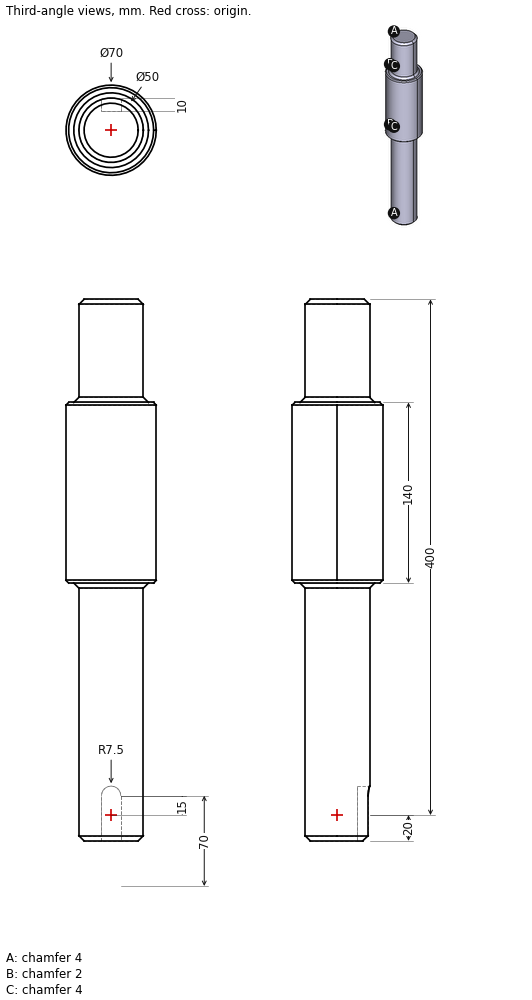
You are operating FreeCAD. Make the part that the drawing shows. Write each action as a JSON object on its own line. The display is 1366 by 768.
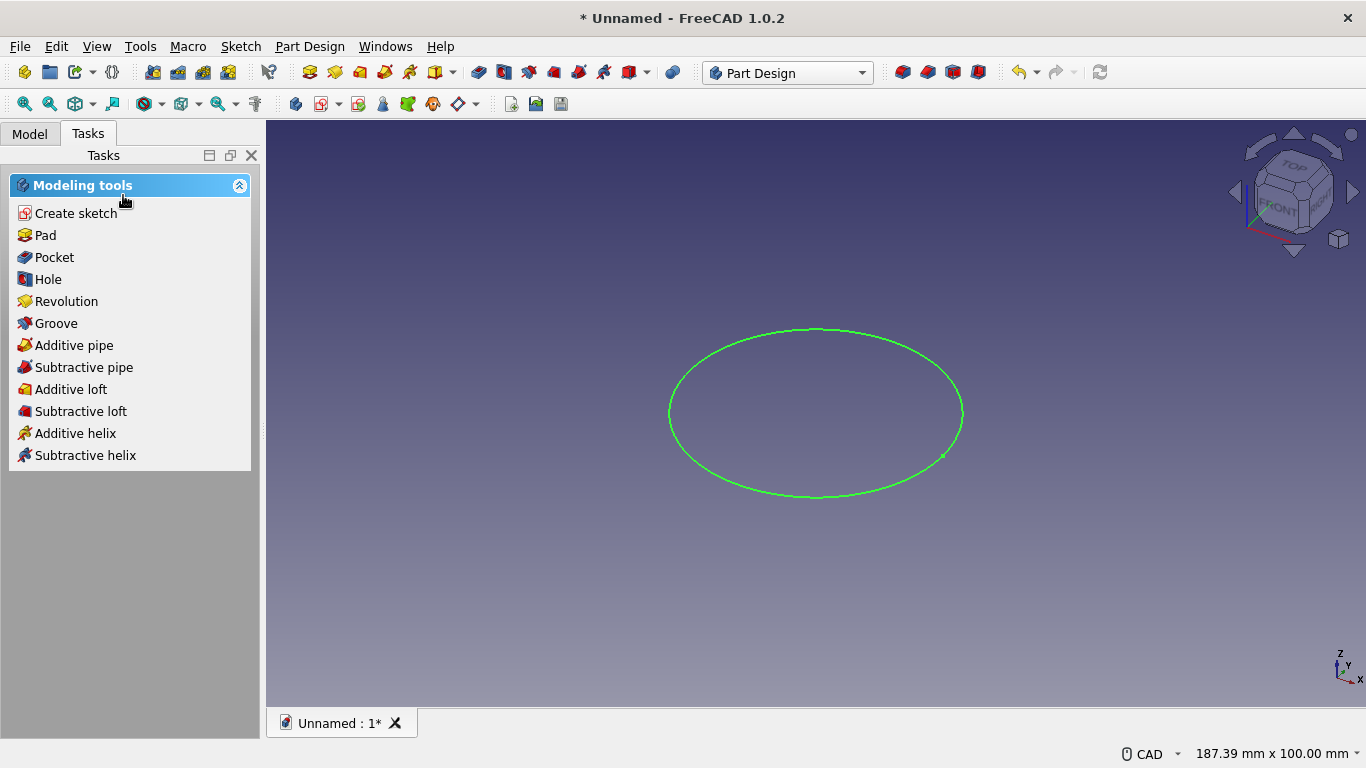
{"action": "left_click", "coordinate": [310, 72]}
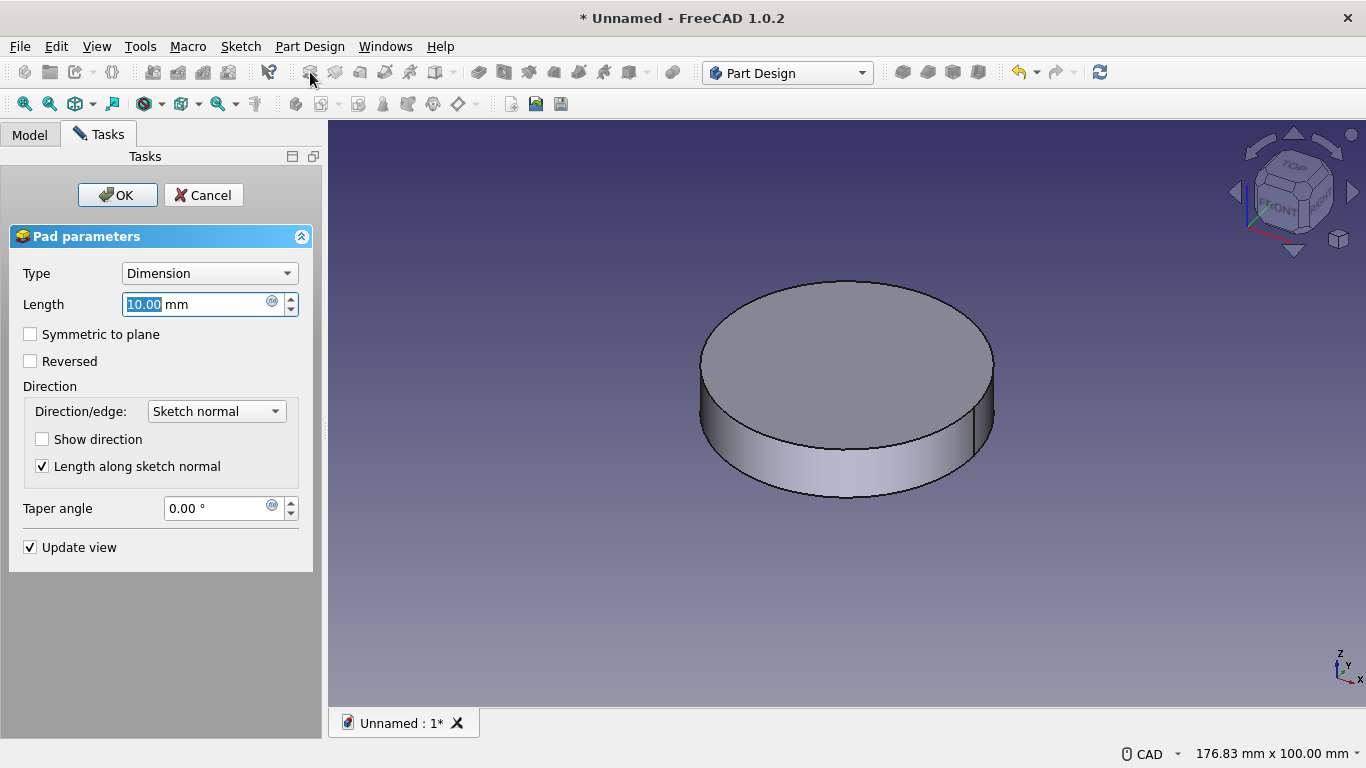
{"action": "left_click", "coordinate": [210, 274]}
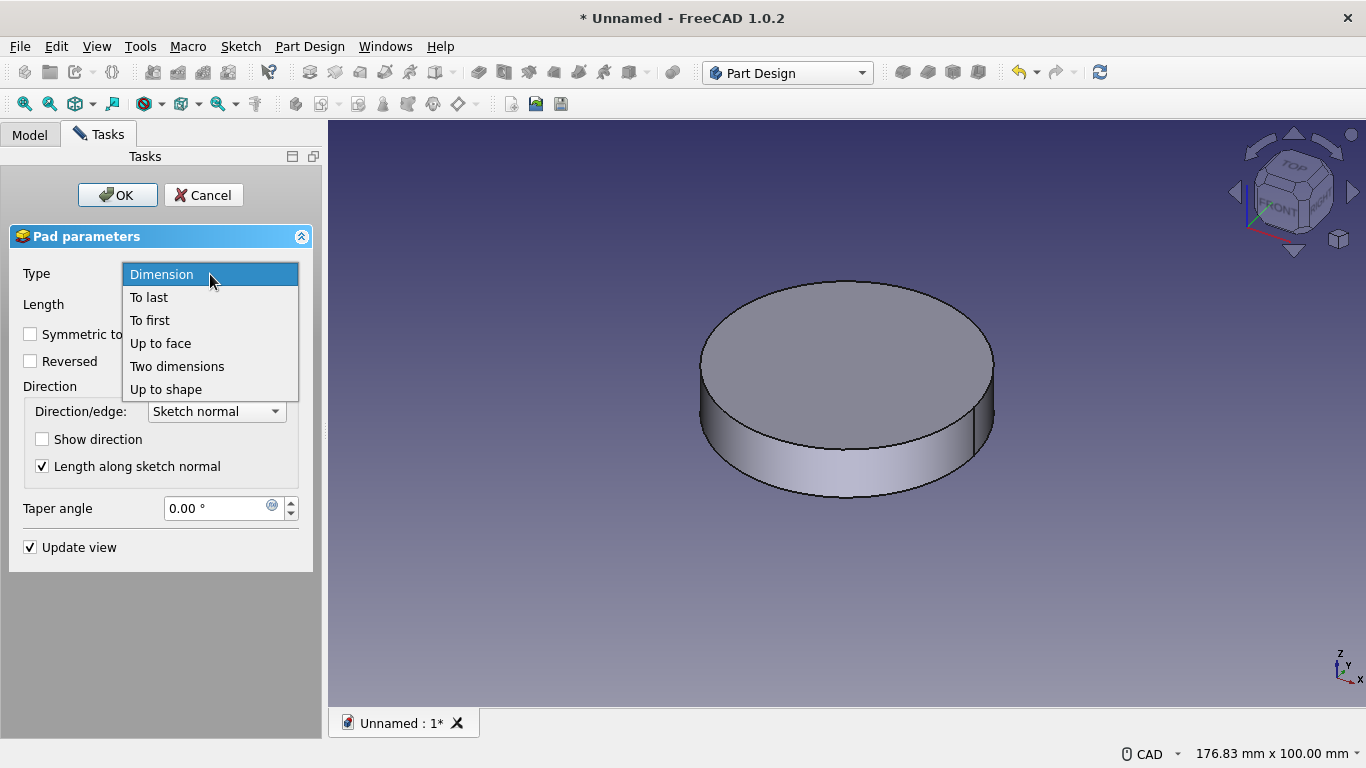
{"action": "left_click", "coordinate": [208, 366]}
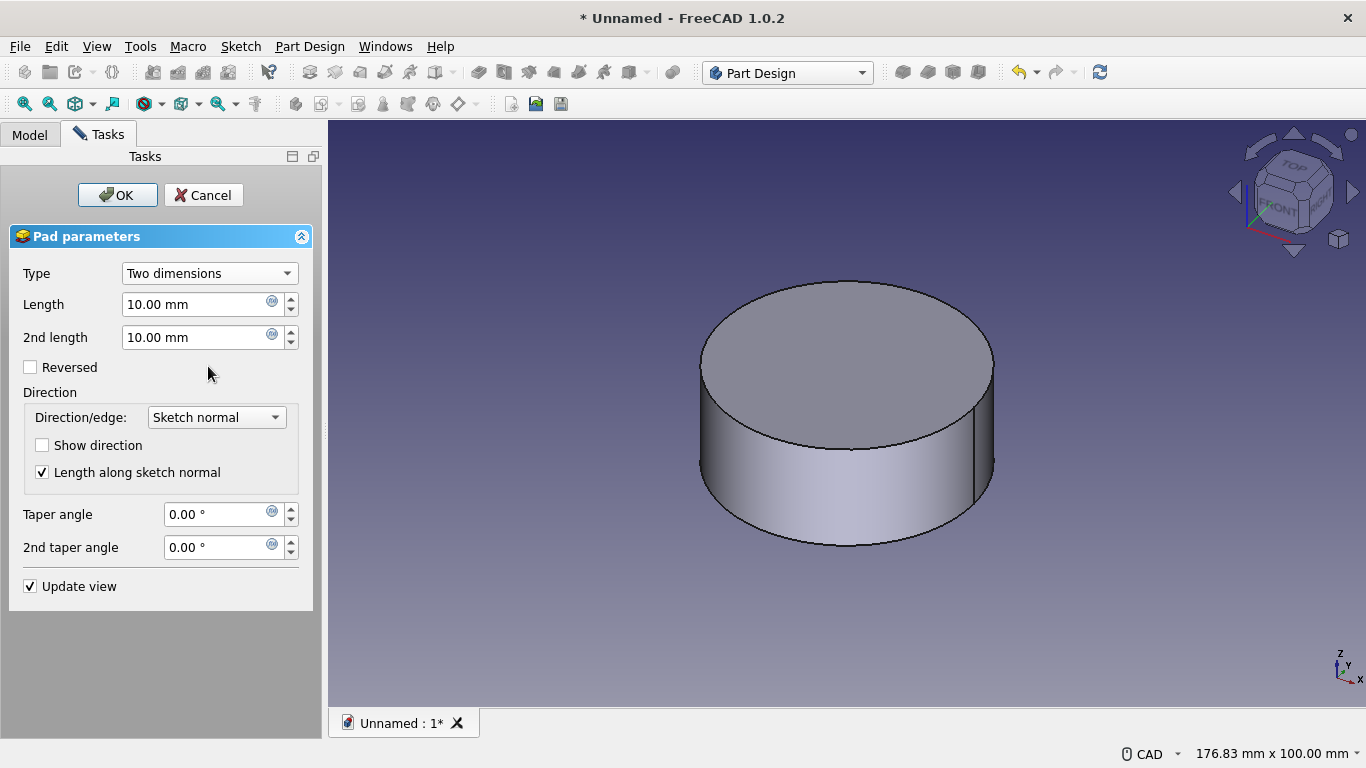
{"action": "triple_click", "coordinate": [204, 304]}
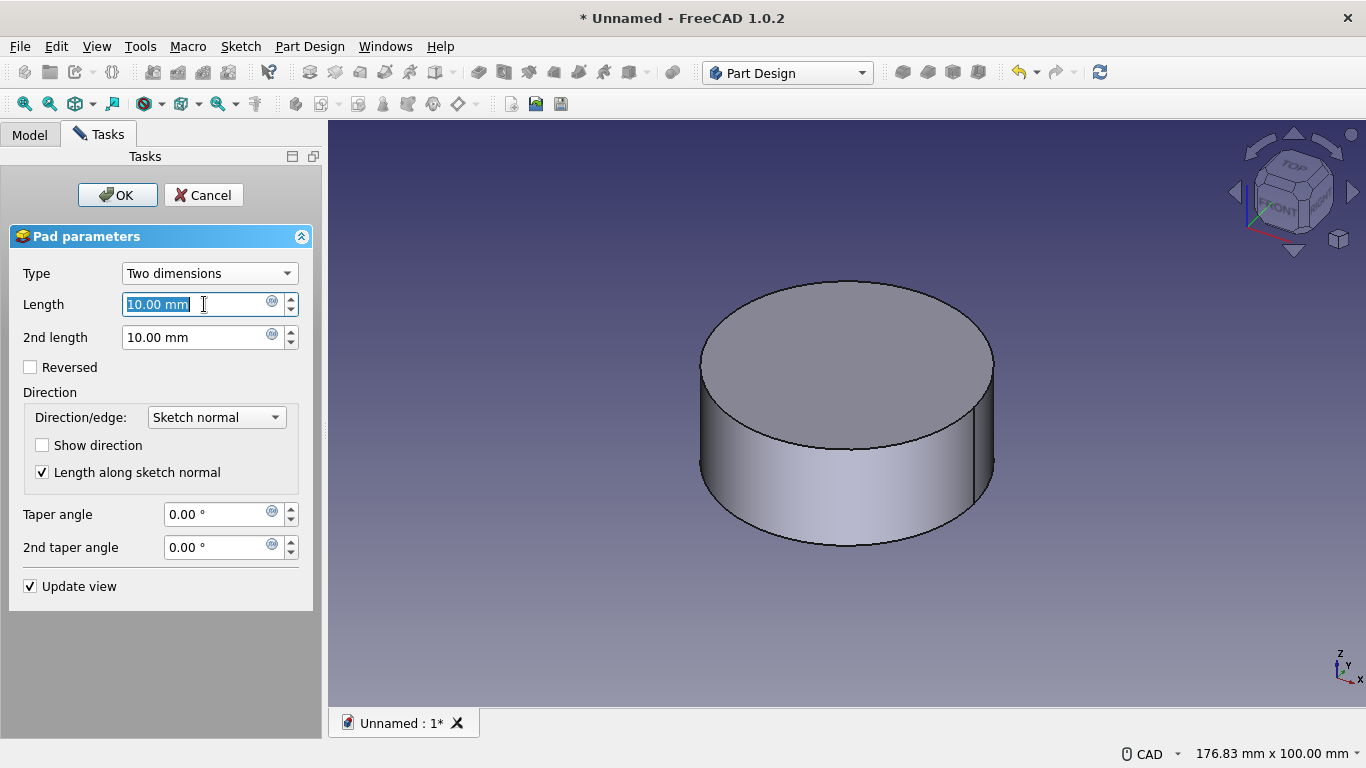
{"action": "type", "text": "400"}
{"action": "key", "text": "Tab"}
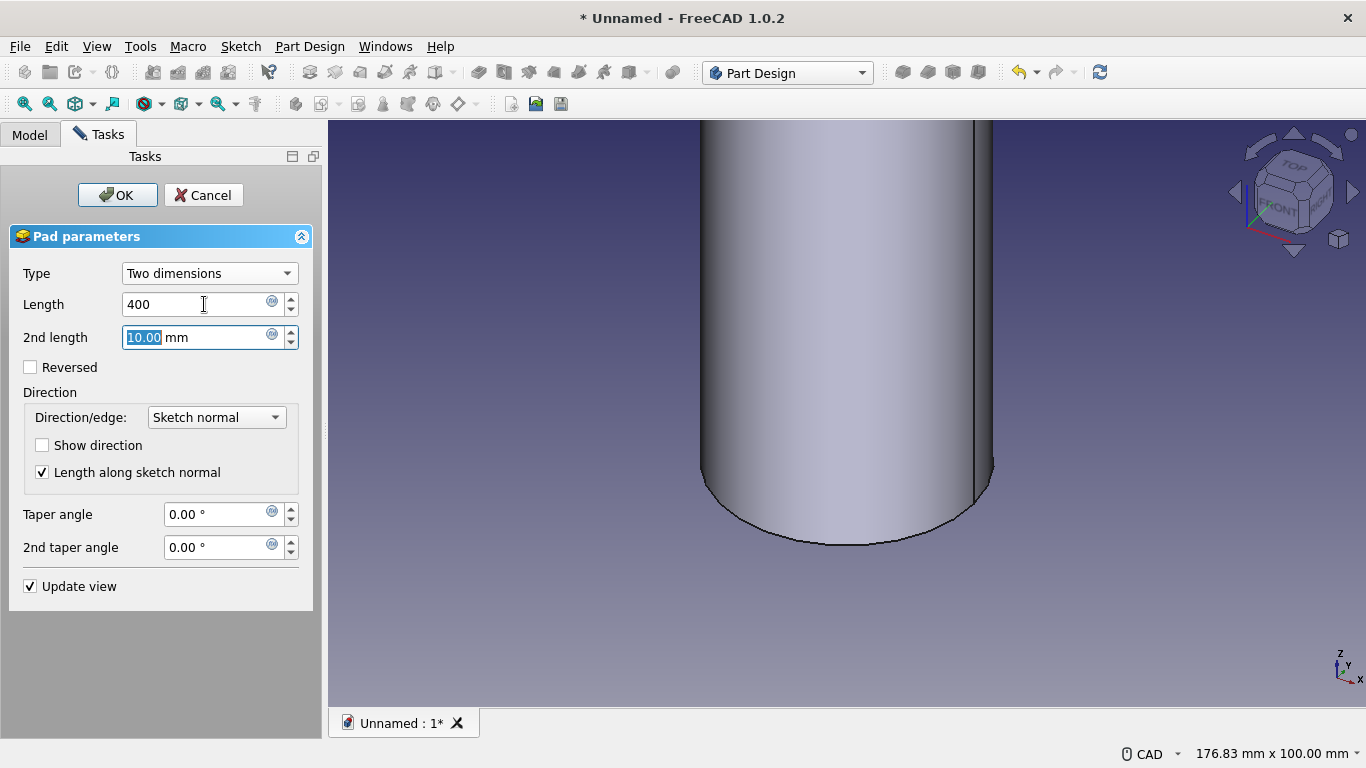
{"action": "type", "text": "20"}
{"action": "key", "text": "Tab"}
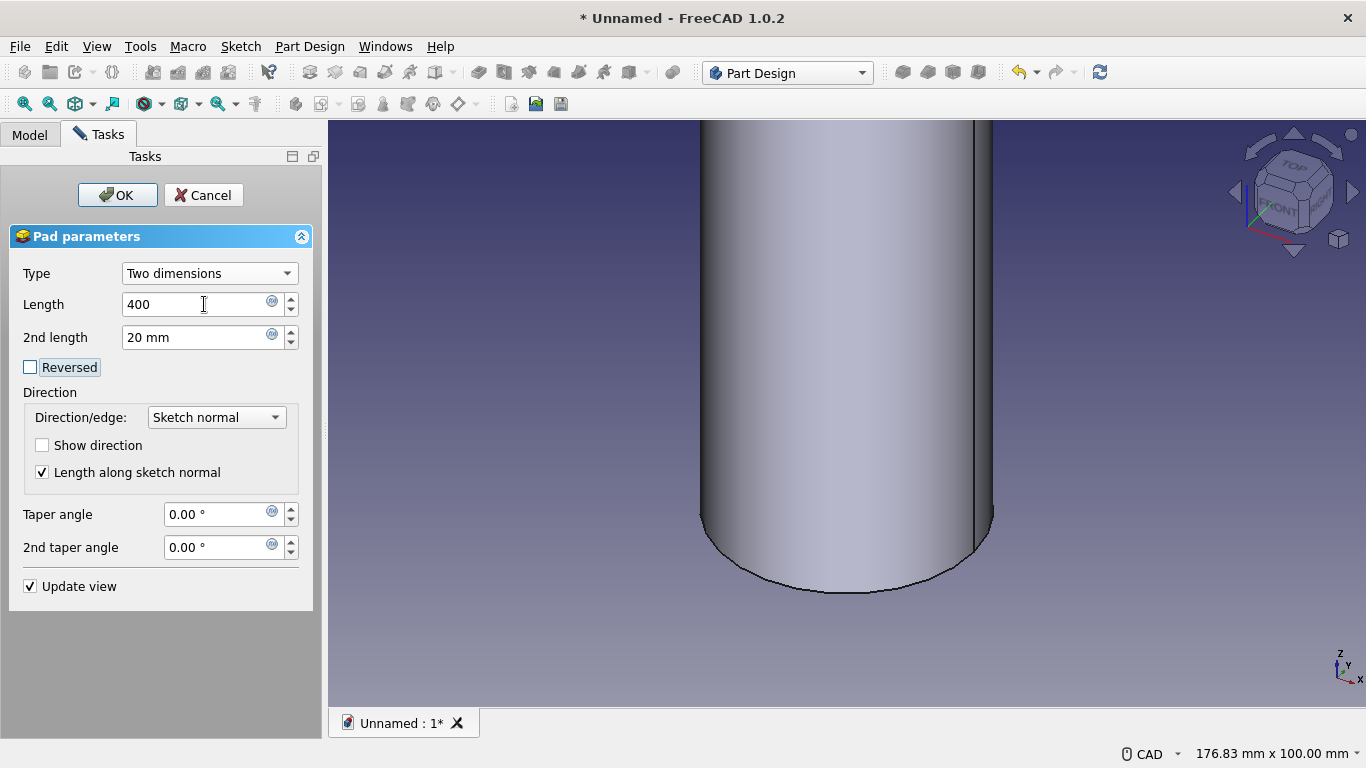
{"action": "left_click", "coordinate": [118, 195]}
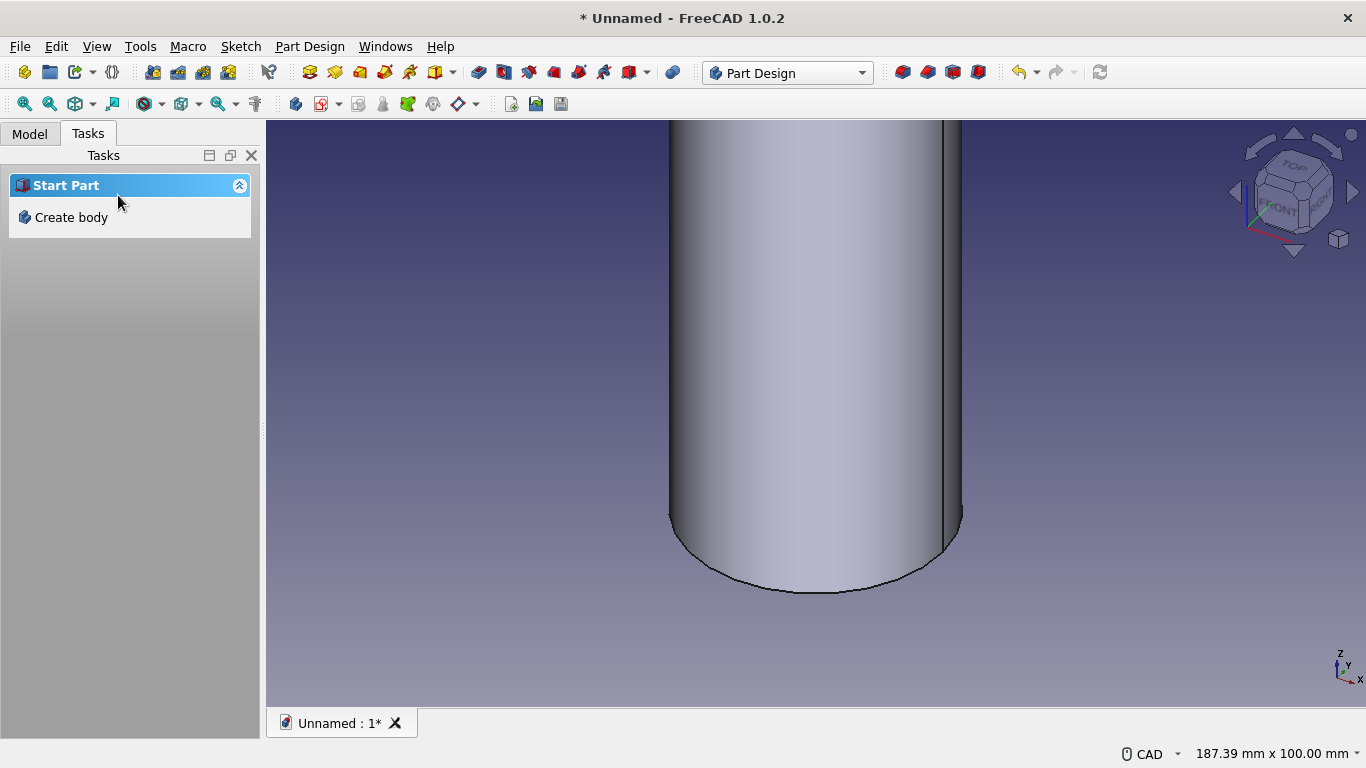
{"action": "left_click", "coordinate": [25, 104]}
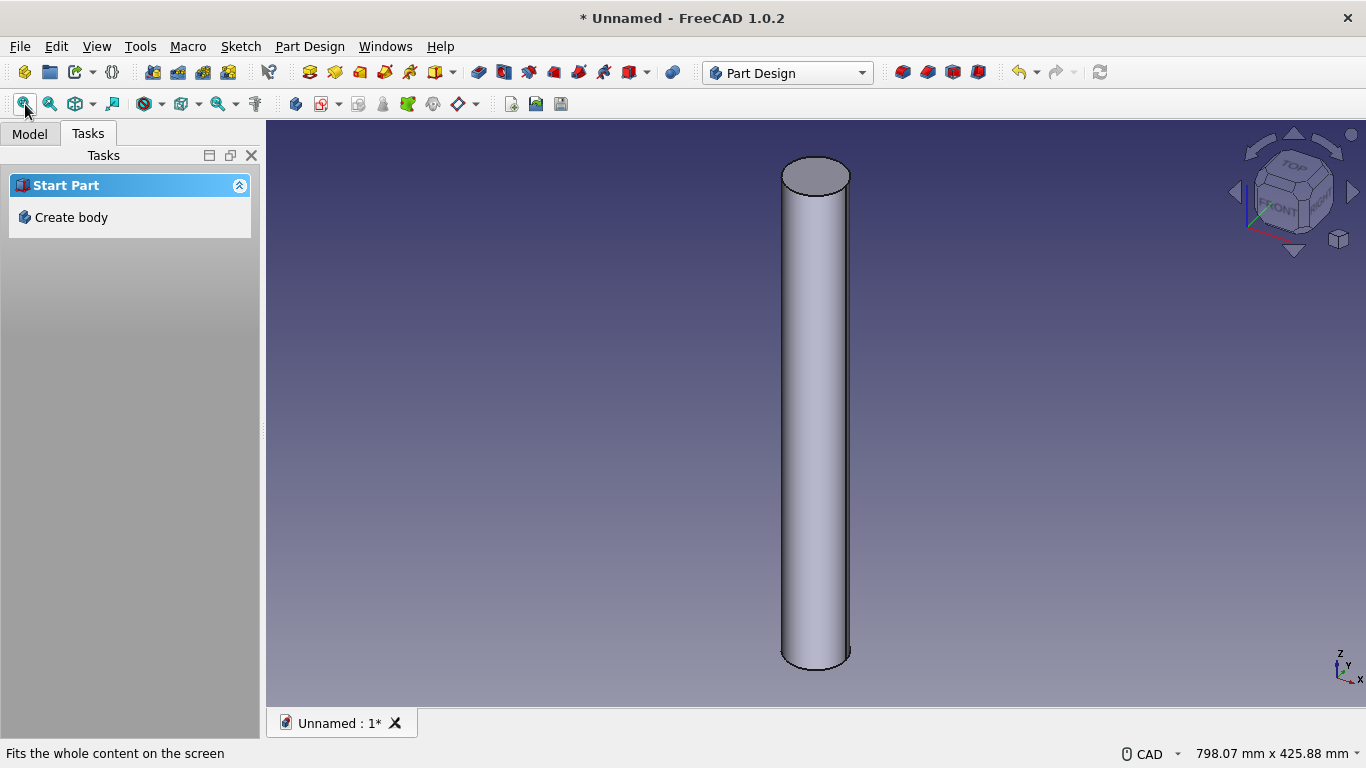
{"action": "left_click", "coordinate": [786, 165]}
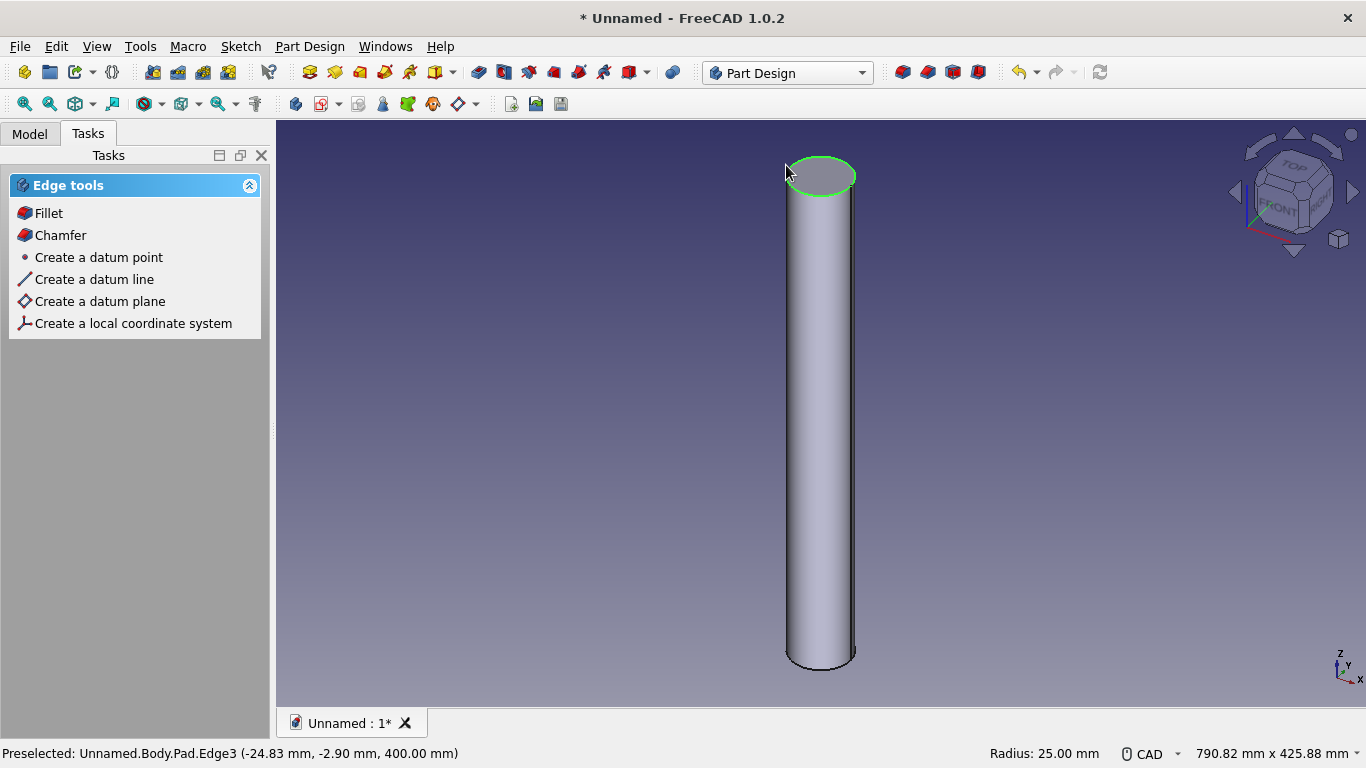
{"action": "key", "text": "0"}